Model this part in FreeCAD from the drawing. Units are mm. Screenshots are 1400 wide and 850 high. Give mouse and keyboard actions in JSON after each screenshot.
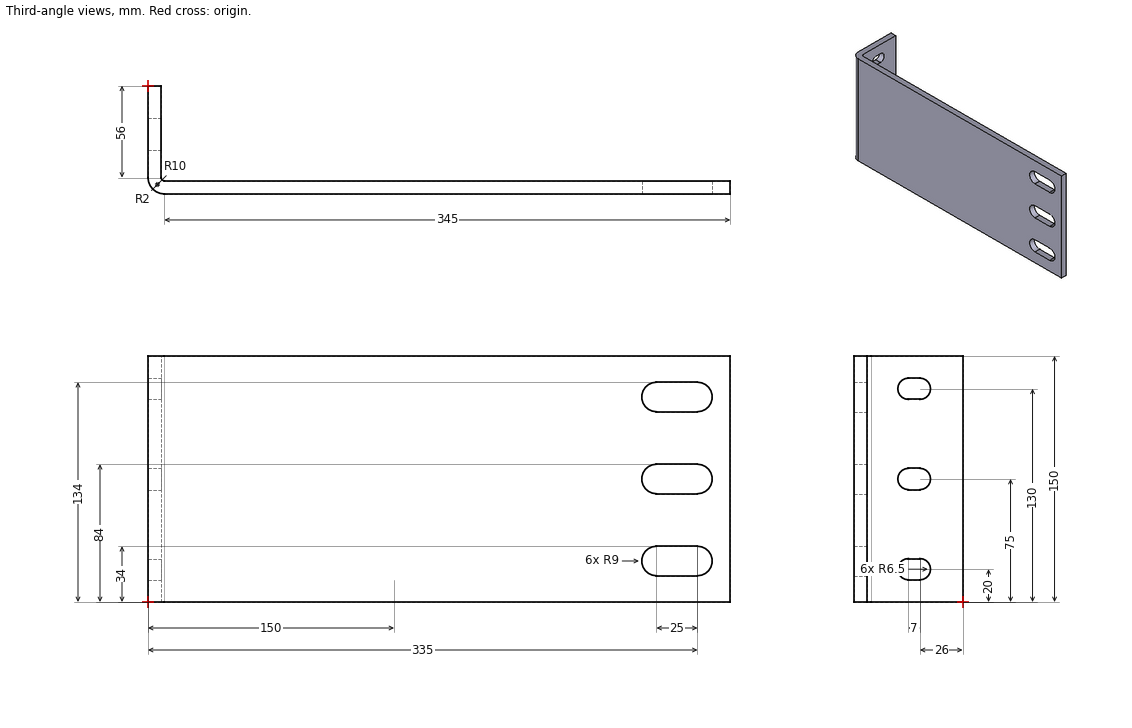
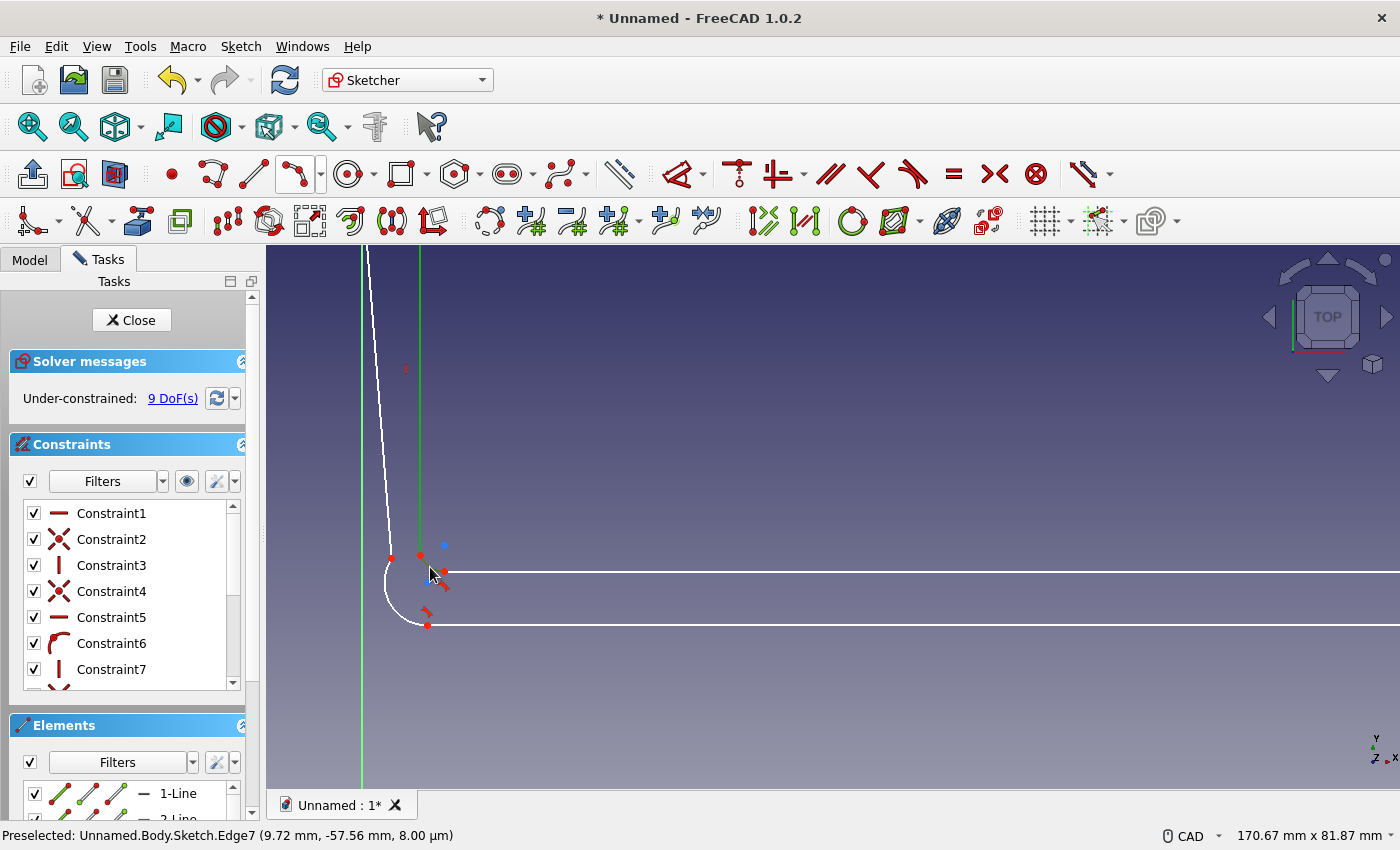
{"action": "left_click", "coordinate": [913, 174]}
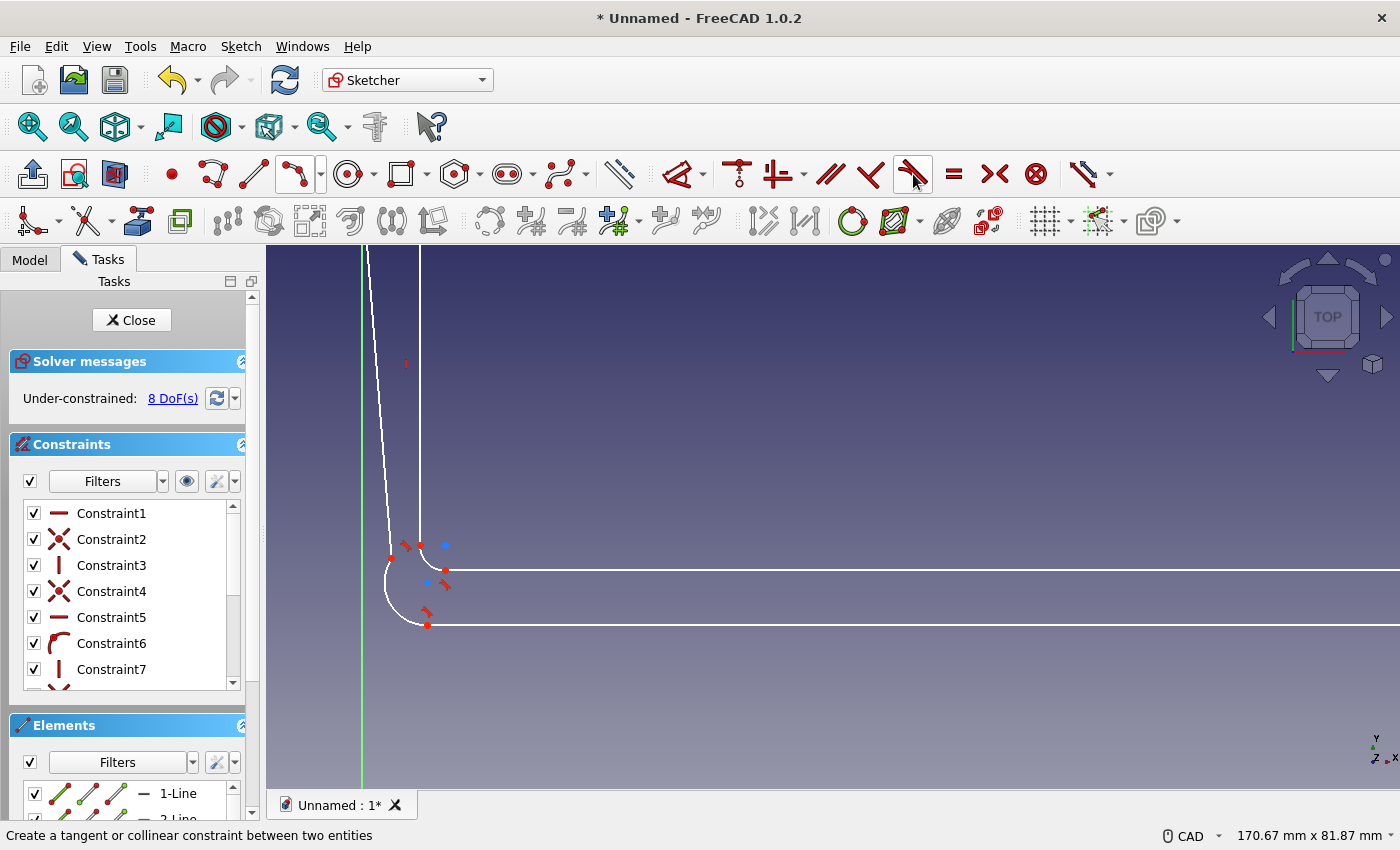
{"action": "left_click", "coordinate": [383, 446]}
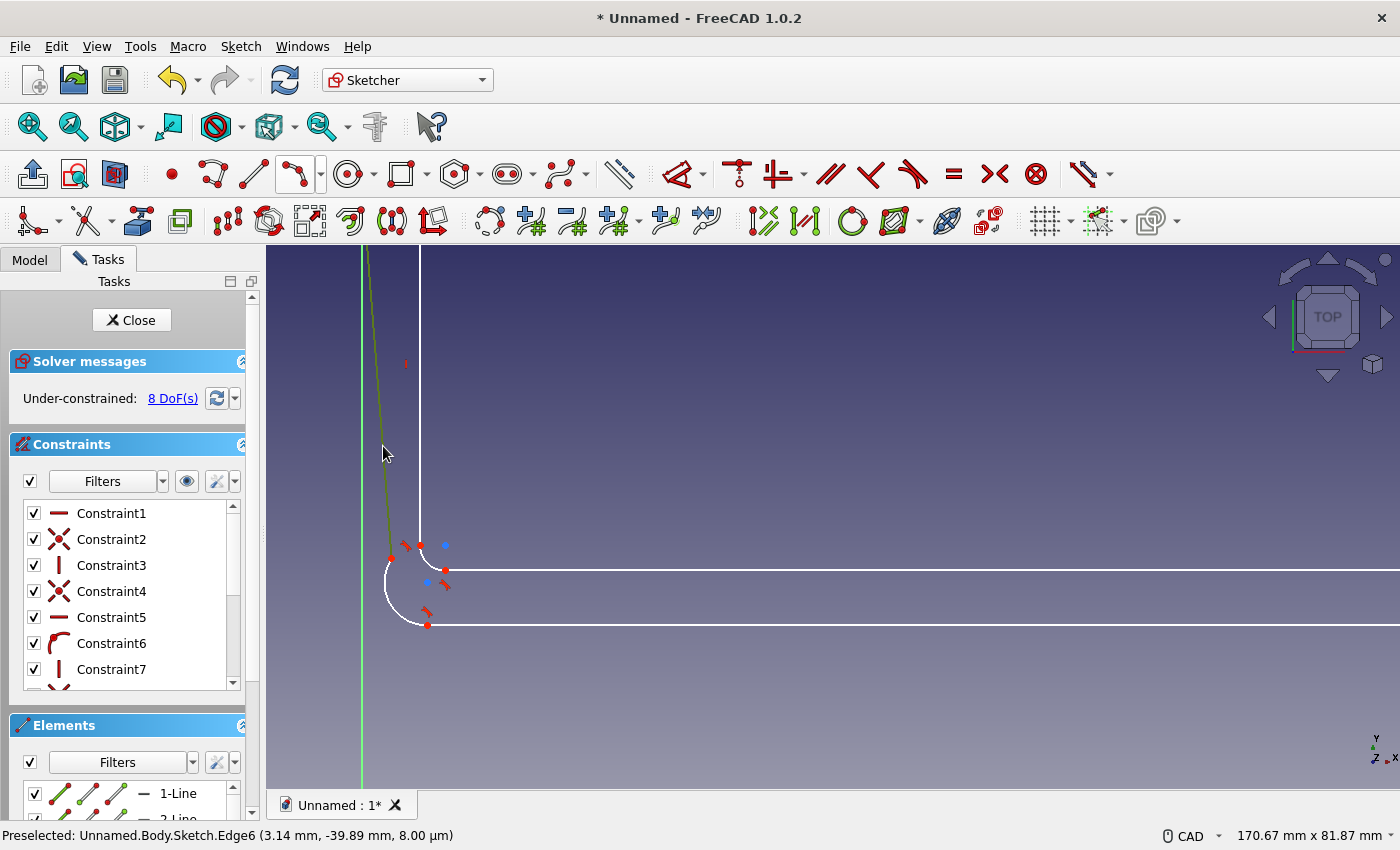
{"action": "left_click", "coordinate": [385, 585]}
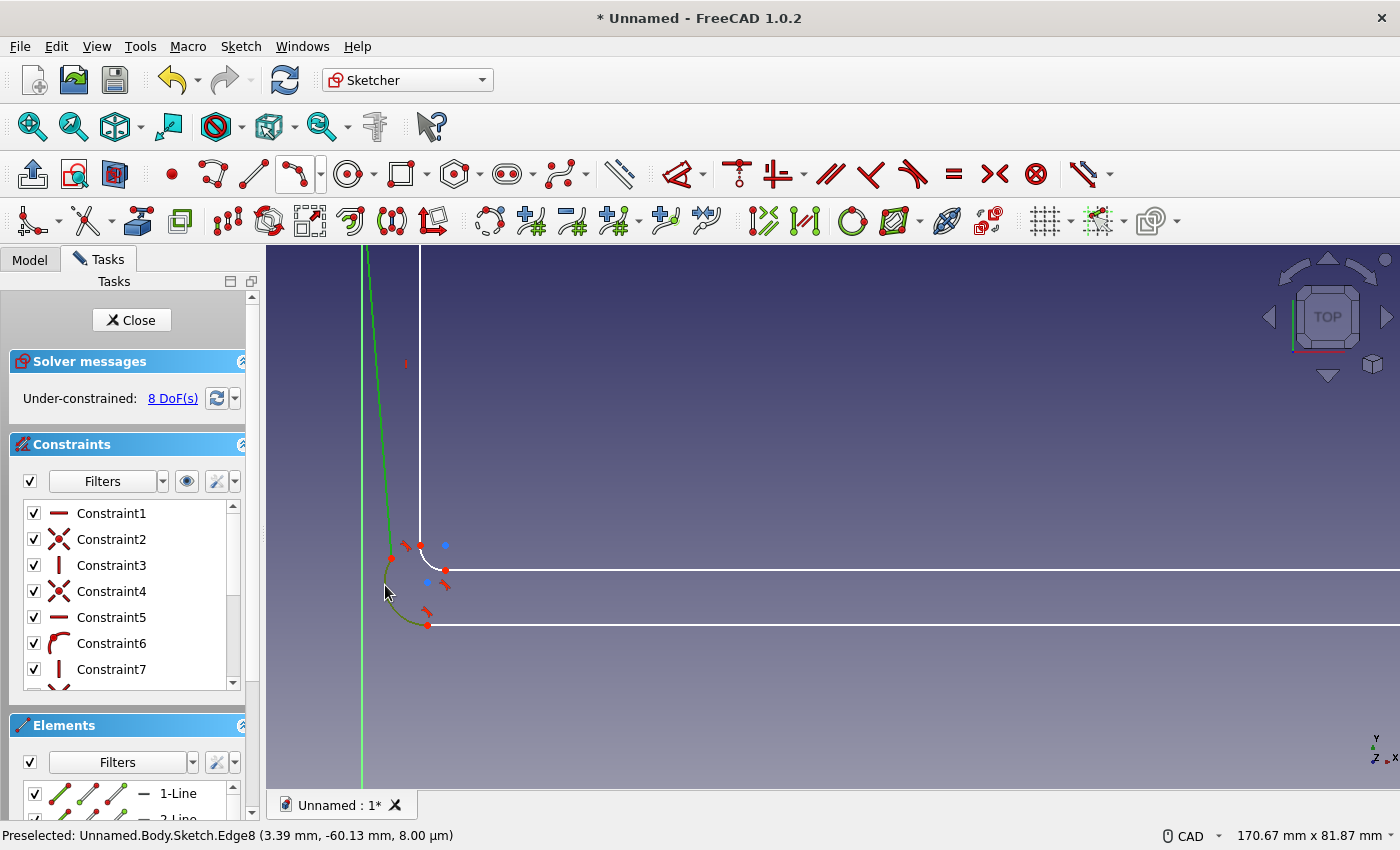
{"action": "left_click", "coordinate": [913, 174]}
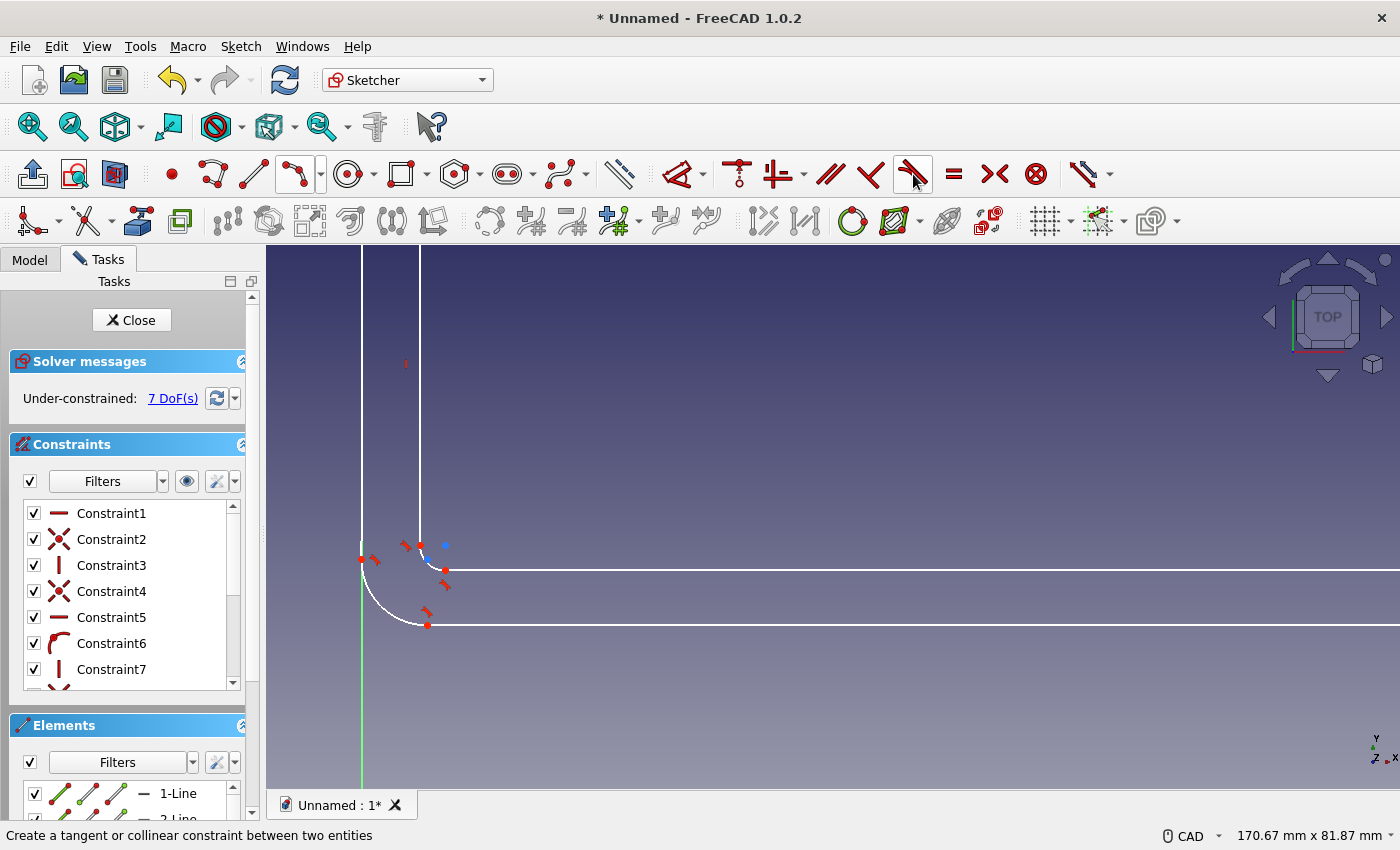
{"action": "left_click", "coordinate": [362, 295]}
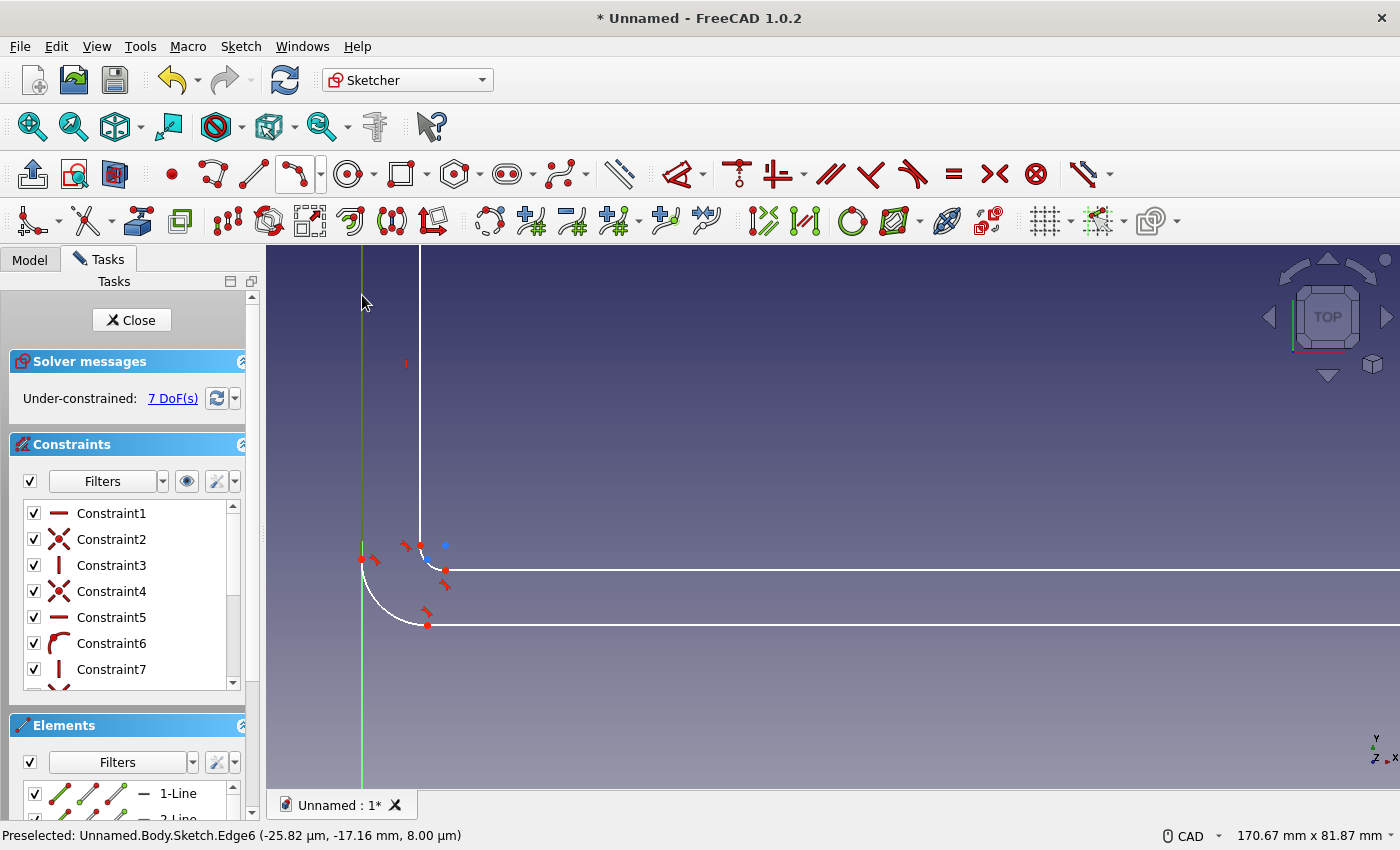
{"action": "left_click", "coordinate": [804, 174]}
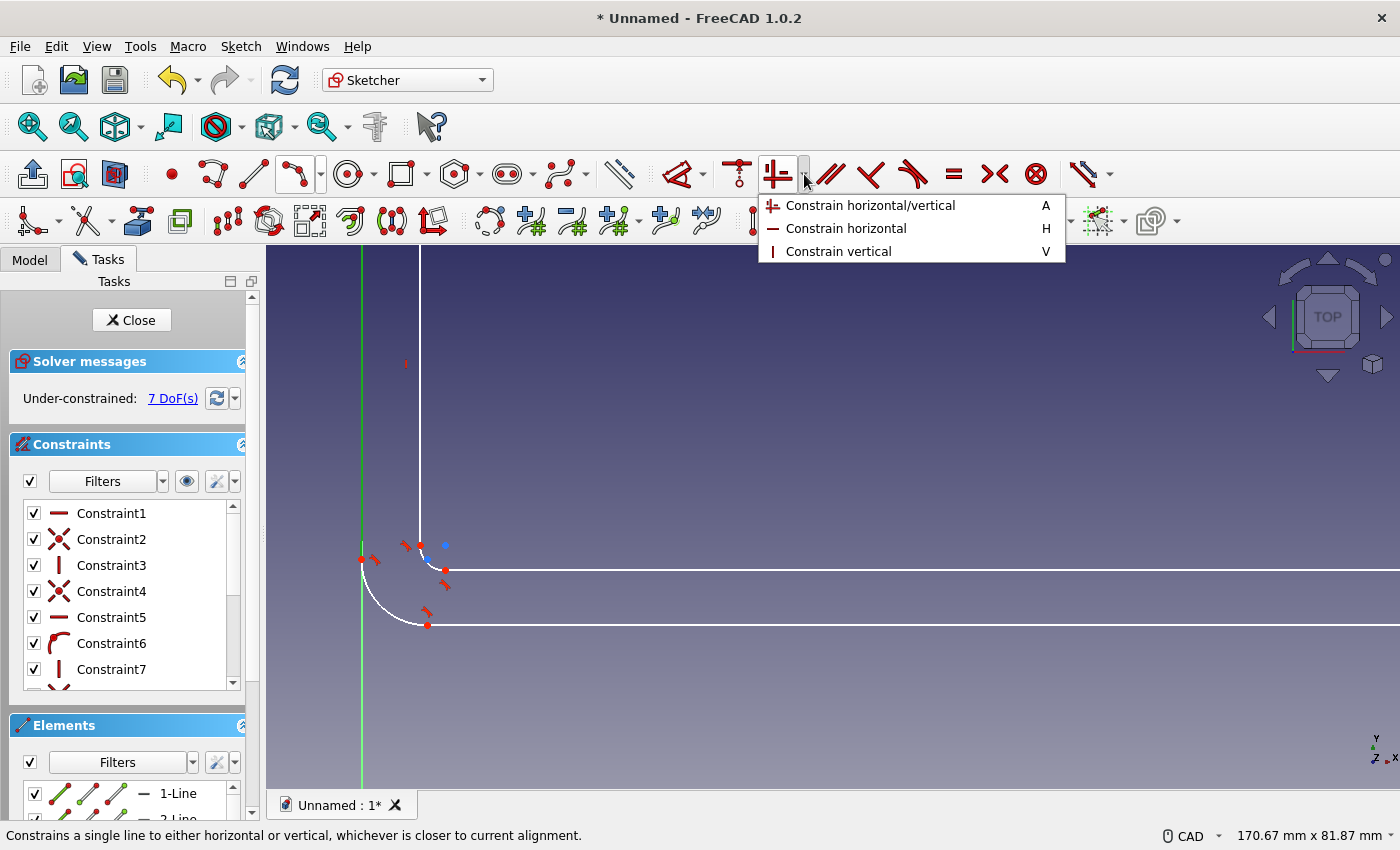
{"action": "left_click", "coordinate": [912, 252]}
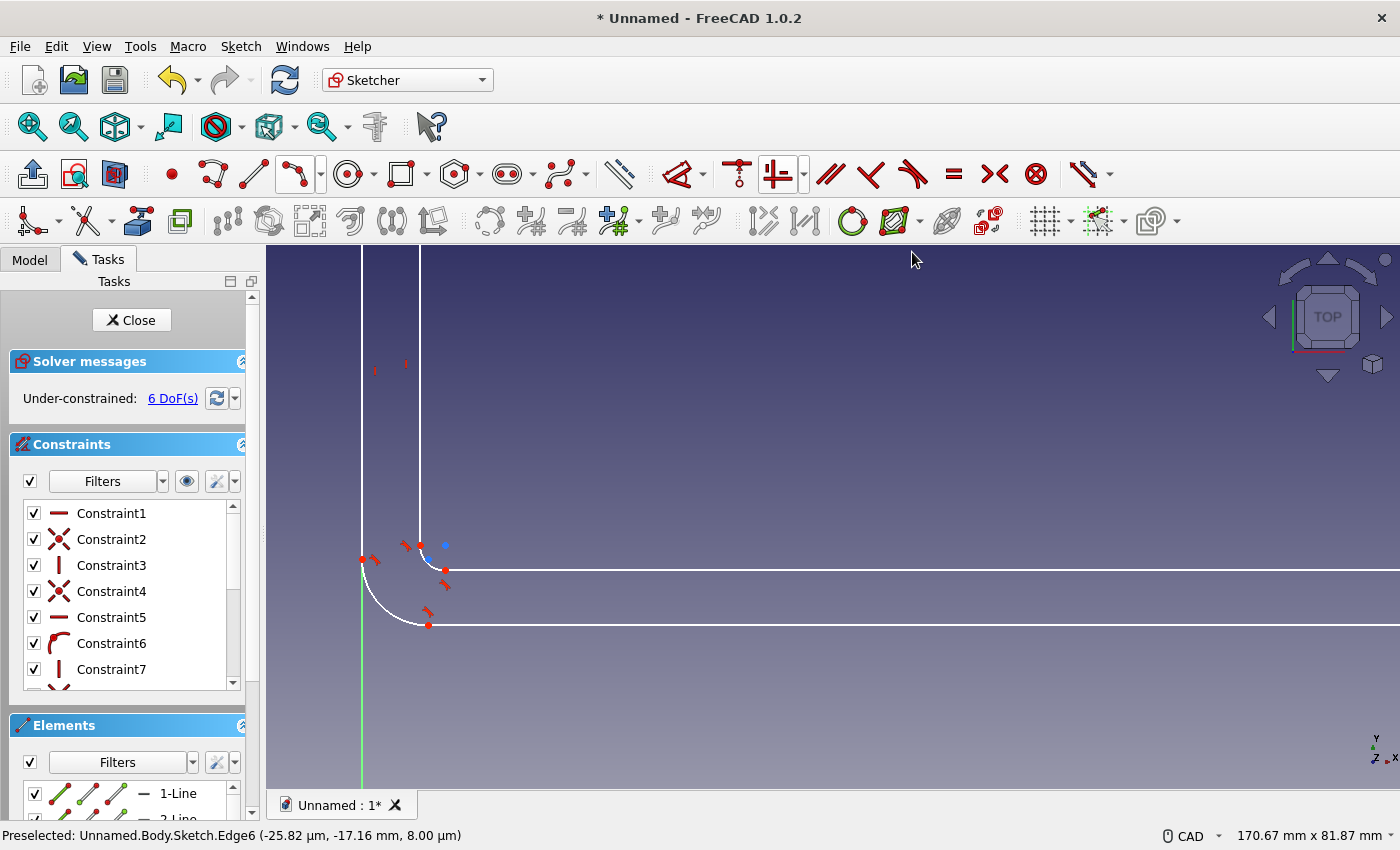
{"action": "left_click", "coordinate": [423, 557]}